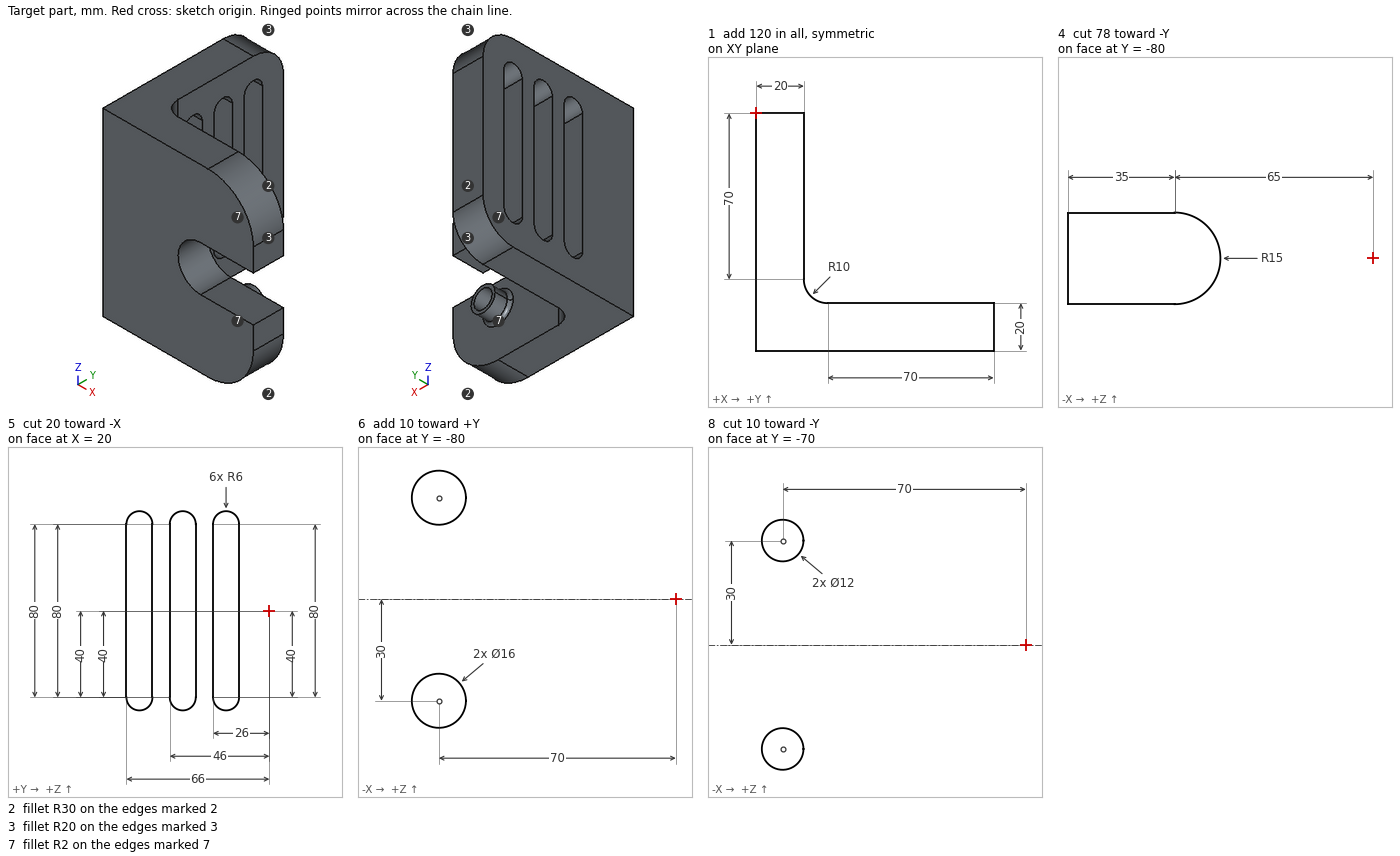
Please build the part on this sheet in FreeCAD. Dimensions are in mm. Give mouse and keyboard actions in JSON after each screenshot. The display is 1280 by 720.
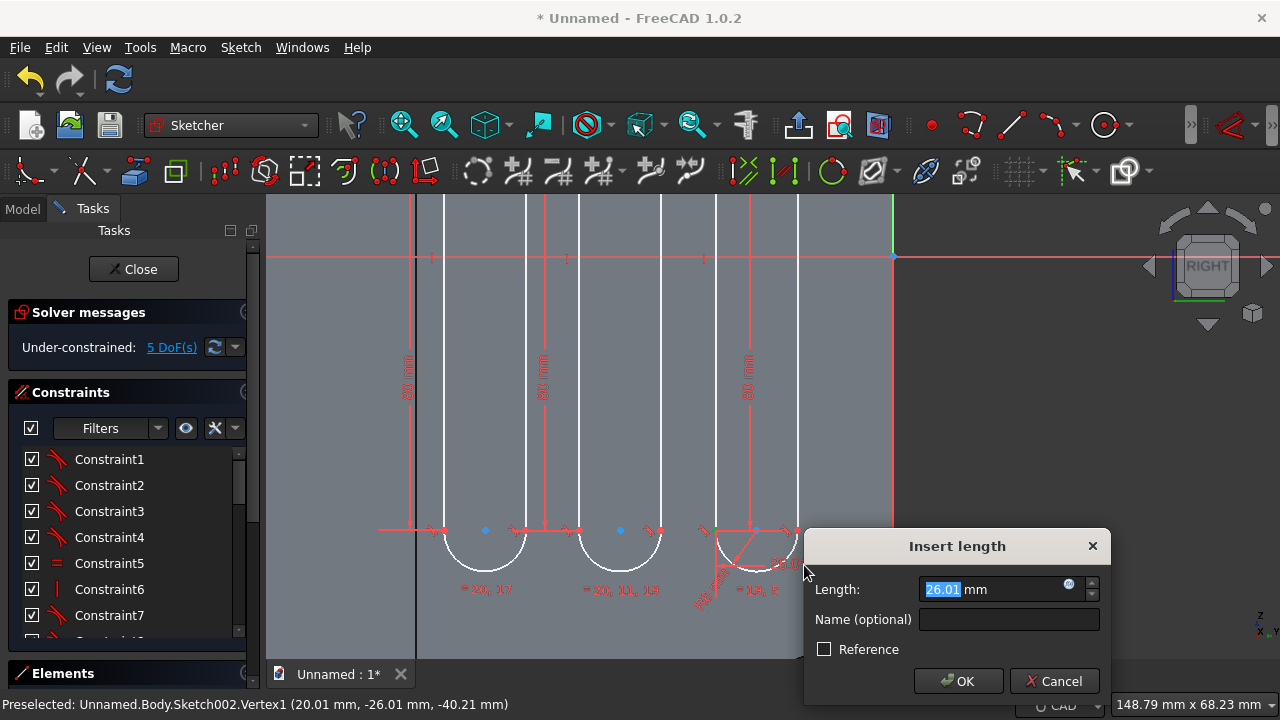
{"action": "type", "text": "26"}
{"action": "key", "text": "Return"}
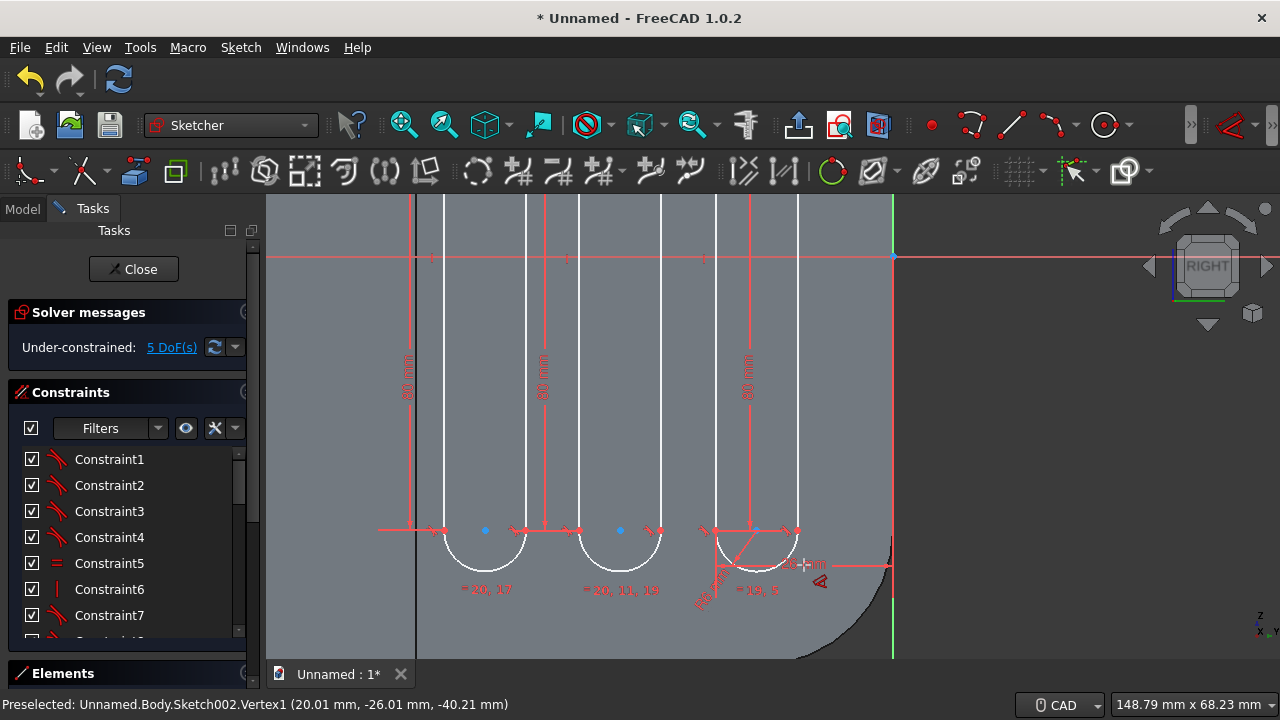
{"action": "left_click", "coordinate": [716, 531]}
{"action": "left_click", "coordinate": [927, 394]}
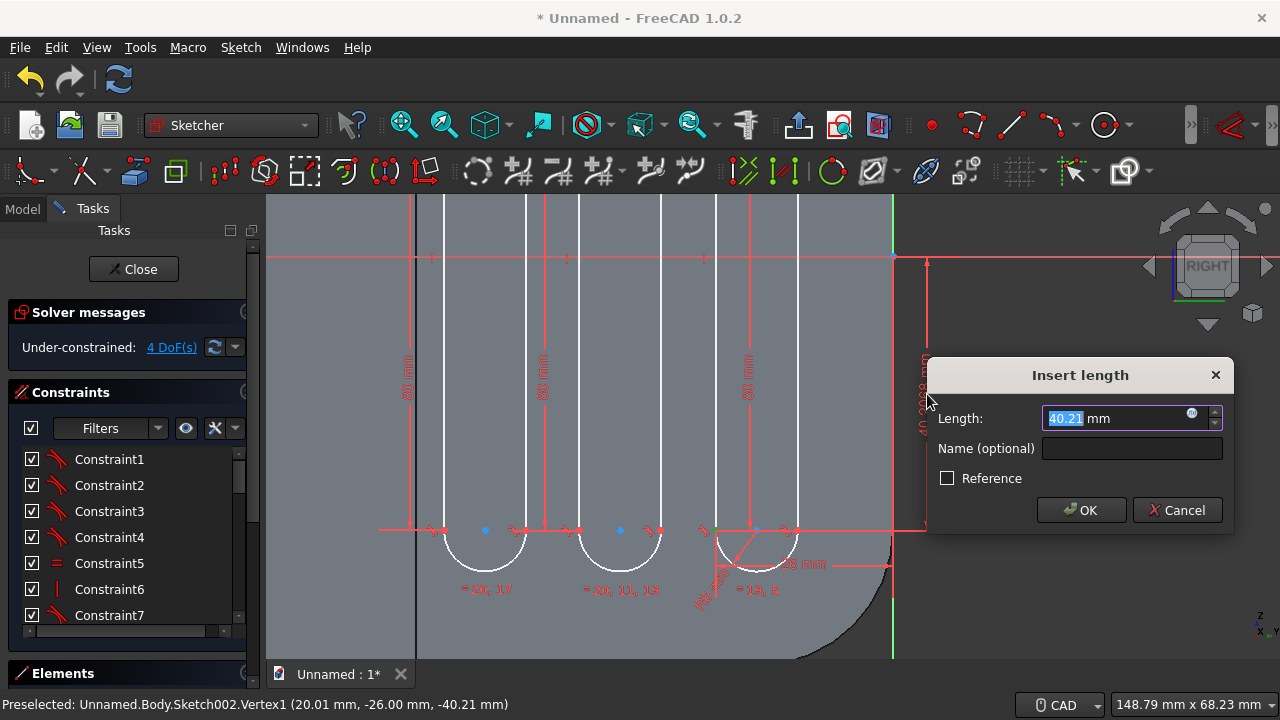
{"action": "type", "text": "40"}
{"action": "key", "text": "Return"}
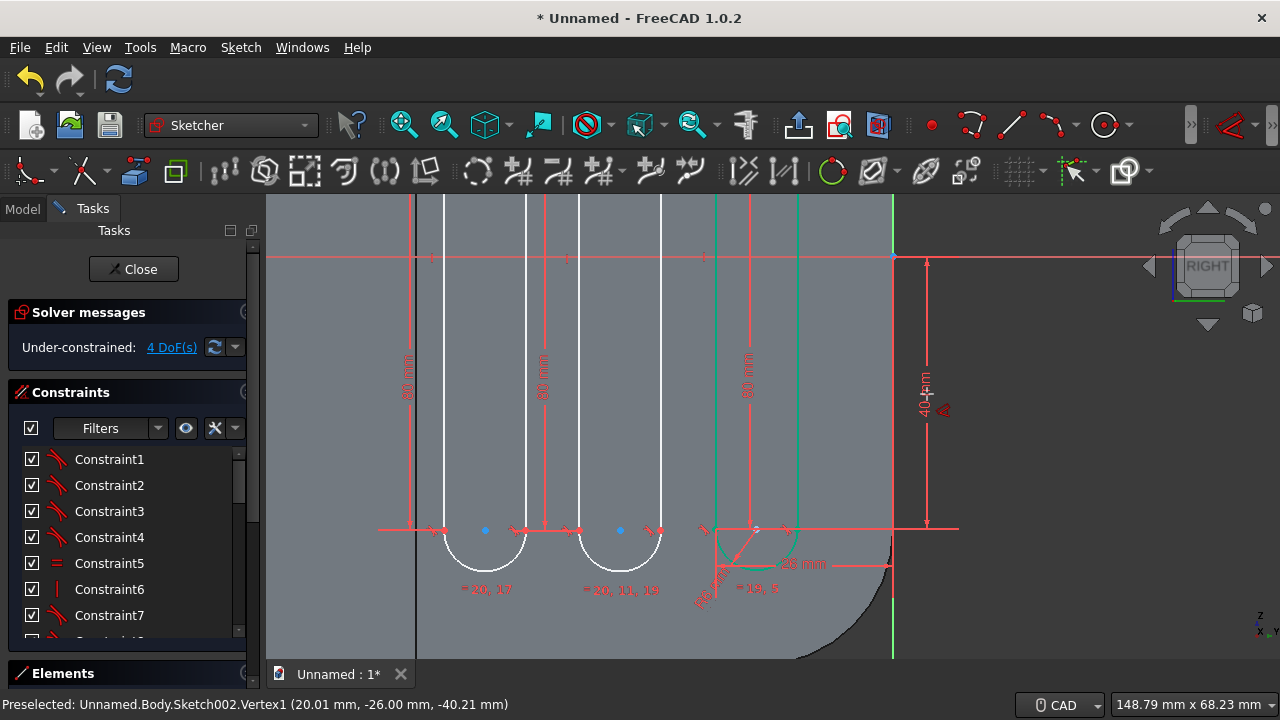
{"action": "left_click", "coordinate": [579, 531]}
{"action": "left_click", "coordinate": [664, 565]}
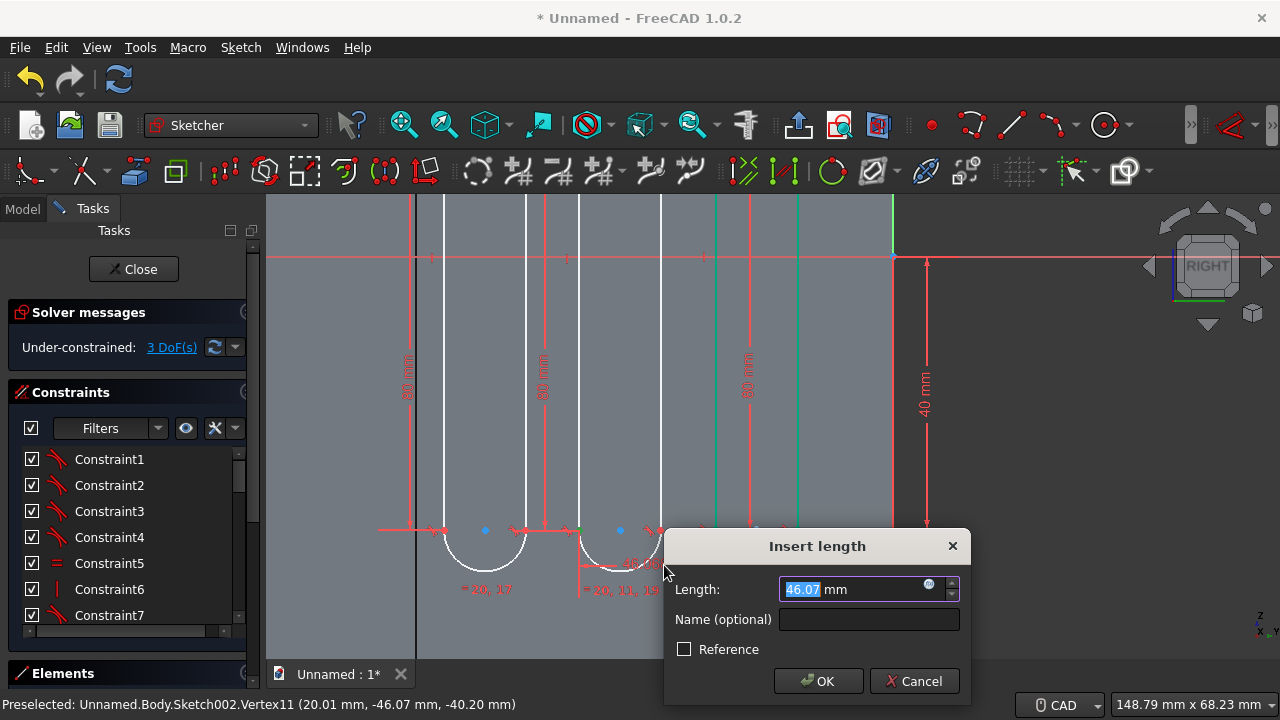
{"action": "type", "text": "46"}
{"action": "key", "text": "Return"}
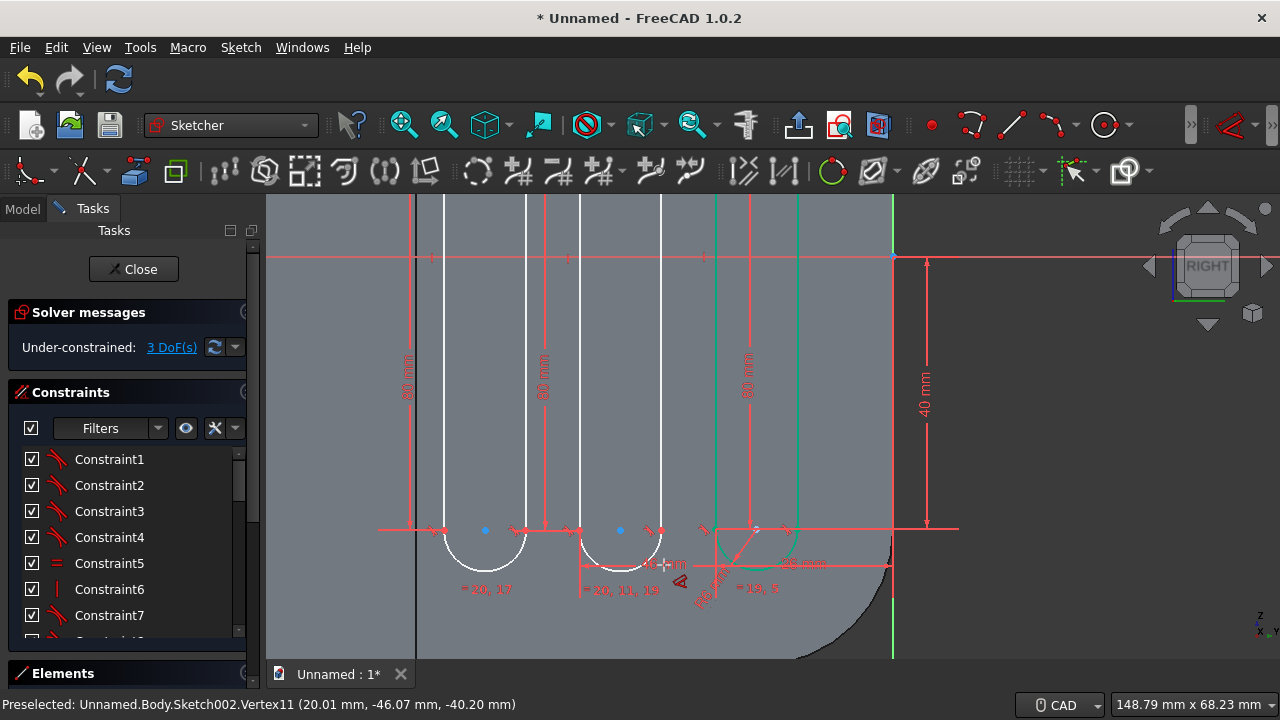
{"action": "left_click", "coordinate": [580, 531]}
{"action": "left_click", "coordinate": [927, 331]}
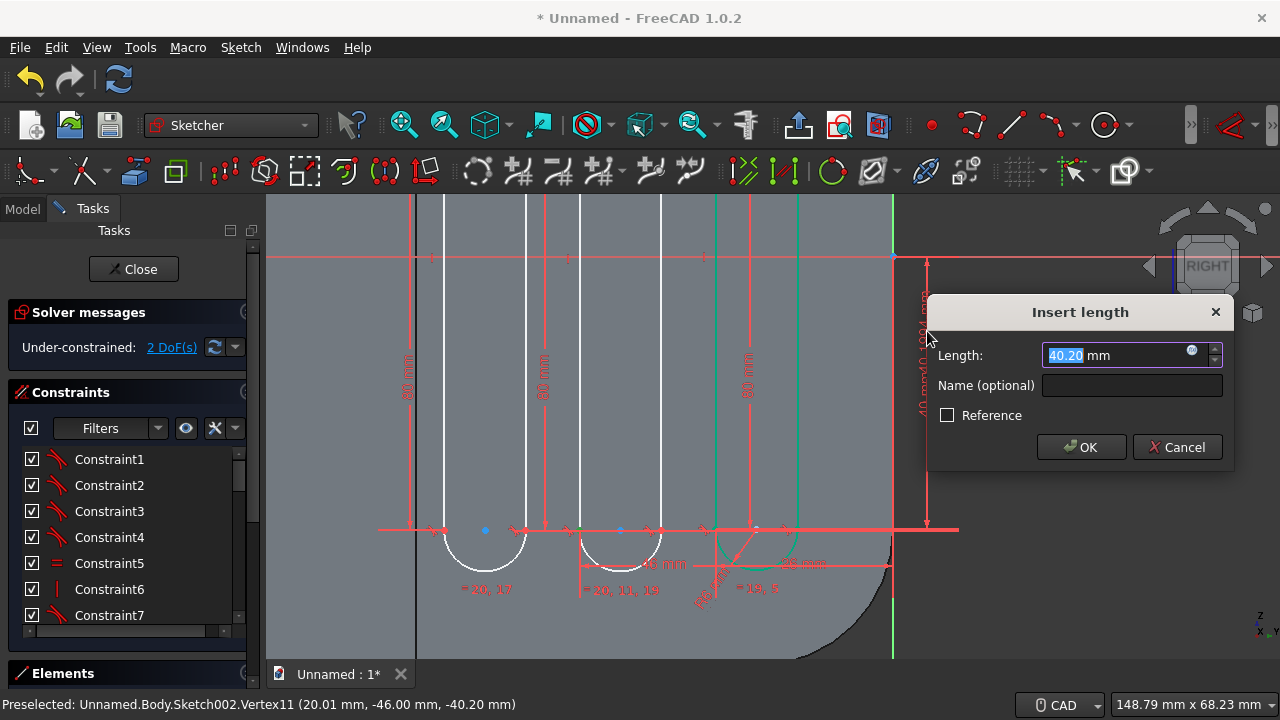
{"action": "type", "text": "40"}
{"action": "key", "text": "Return"}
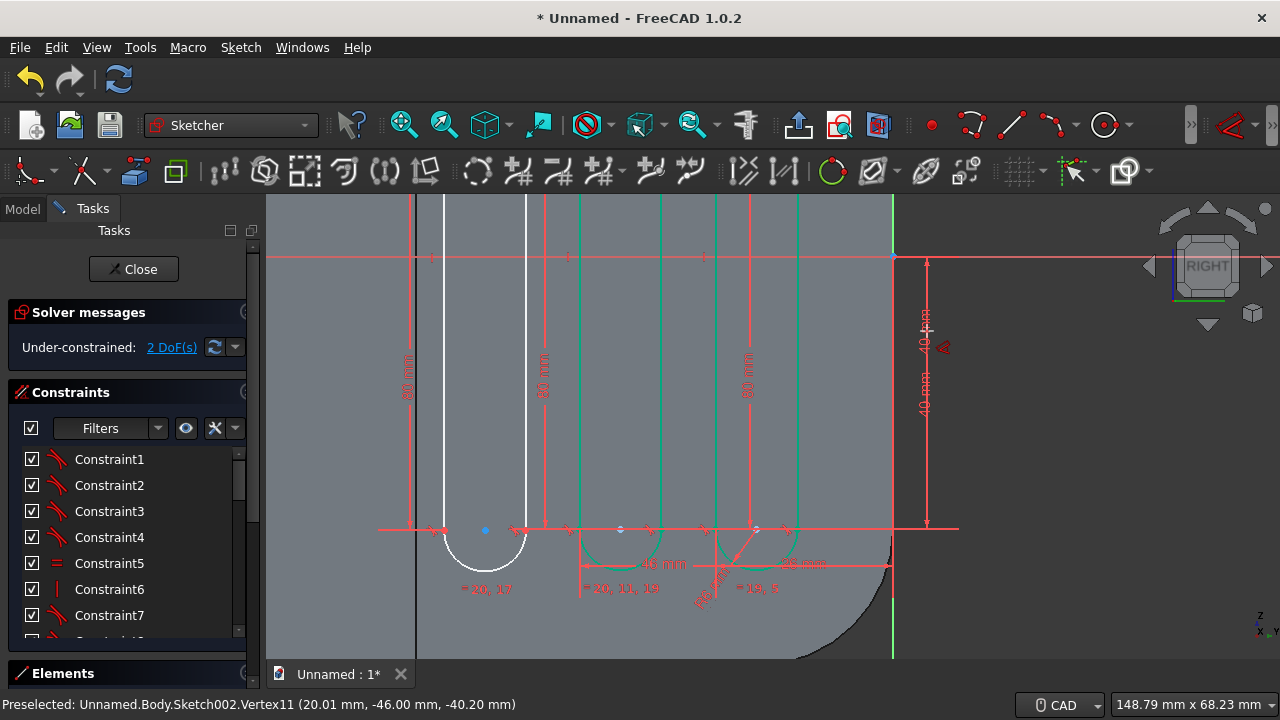
{"action": "left_click", "coordinate": [444, 530]}
{"action": "left_click", "coordinate": [565, 564]}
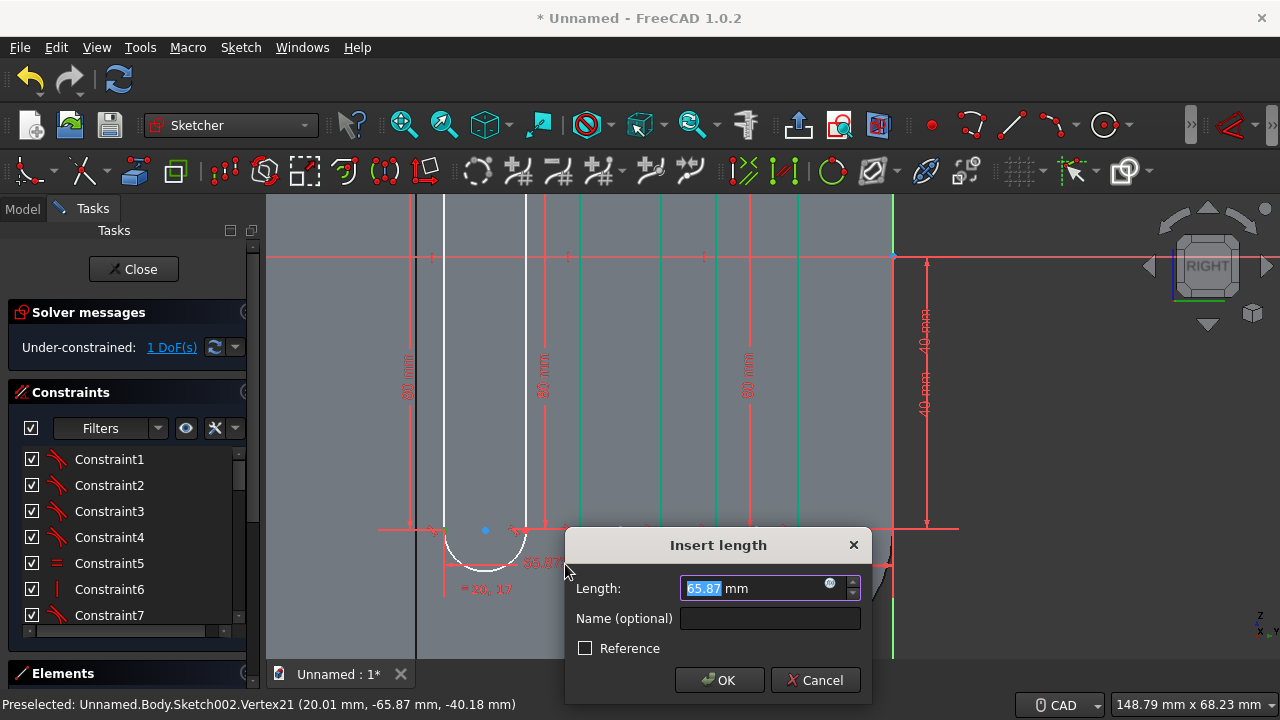
{"action": "type", "text": "66"}
{"action": "key", "text": "Return"}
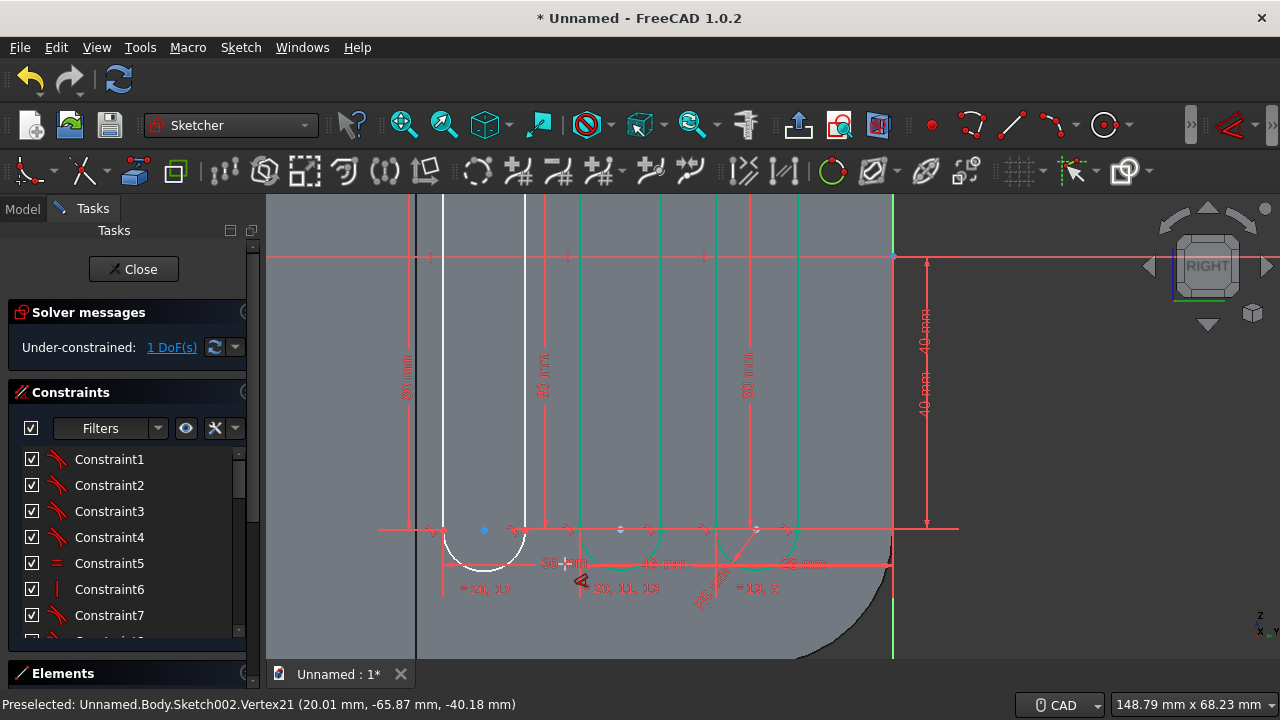
{"action": "left_click", "coordinate": [443, 530]}
{"action": "left_click", "coordinate": [927, 457]}